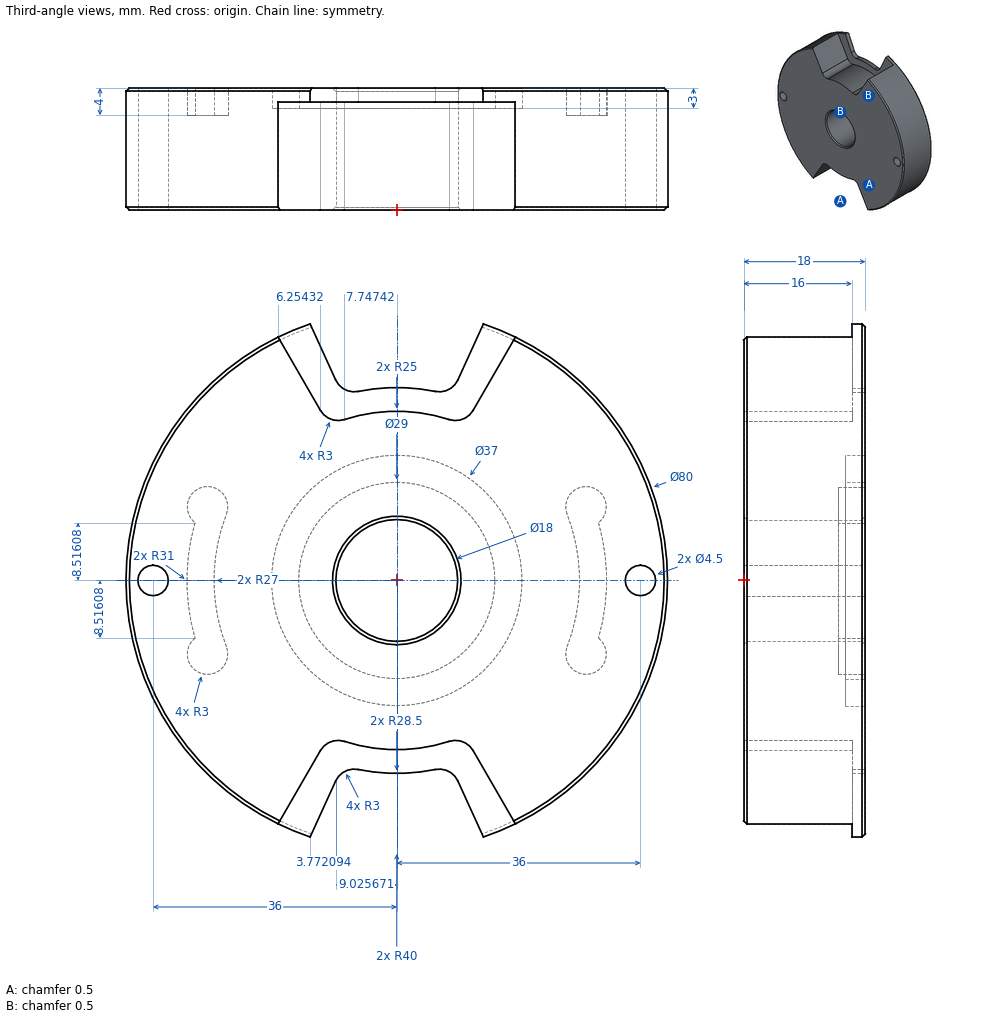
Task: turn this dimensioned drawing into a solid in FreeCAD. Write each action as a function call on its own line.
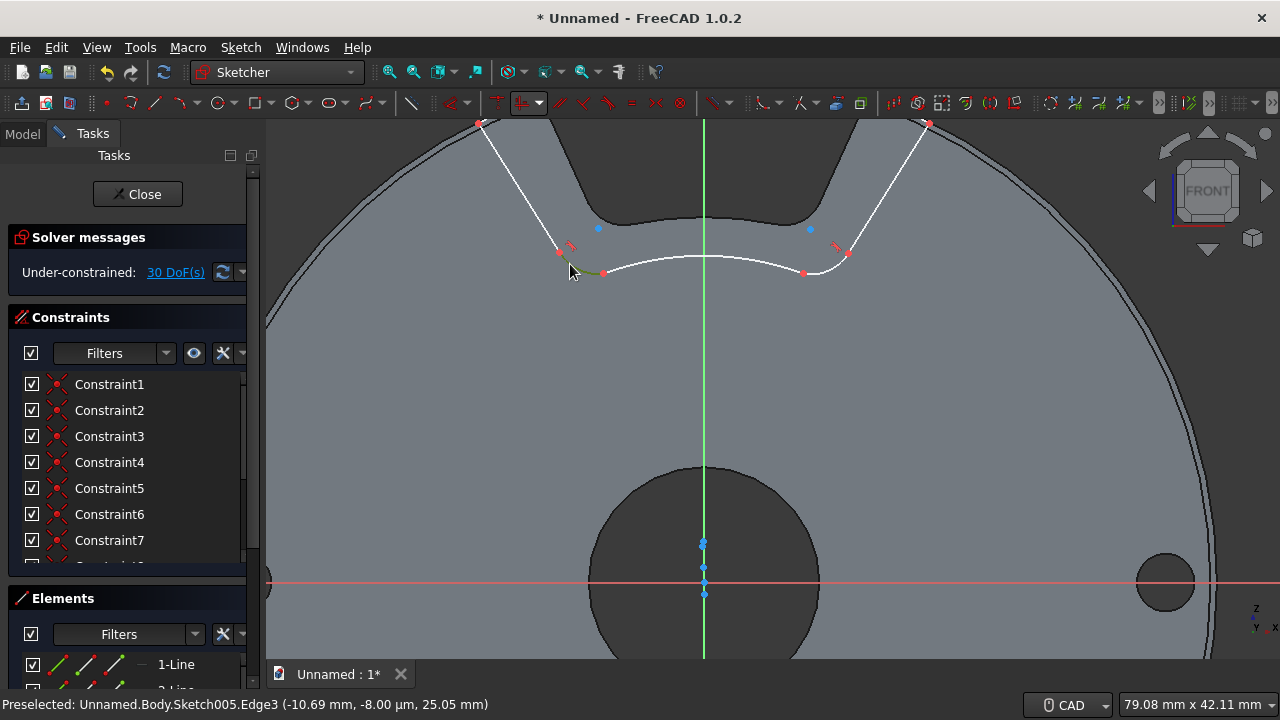
click(744, 259)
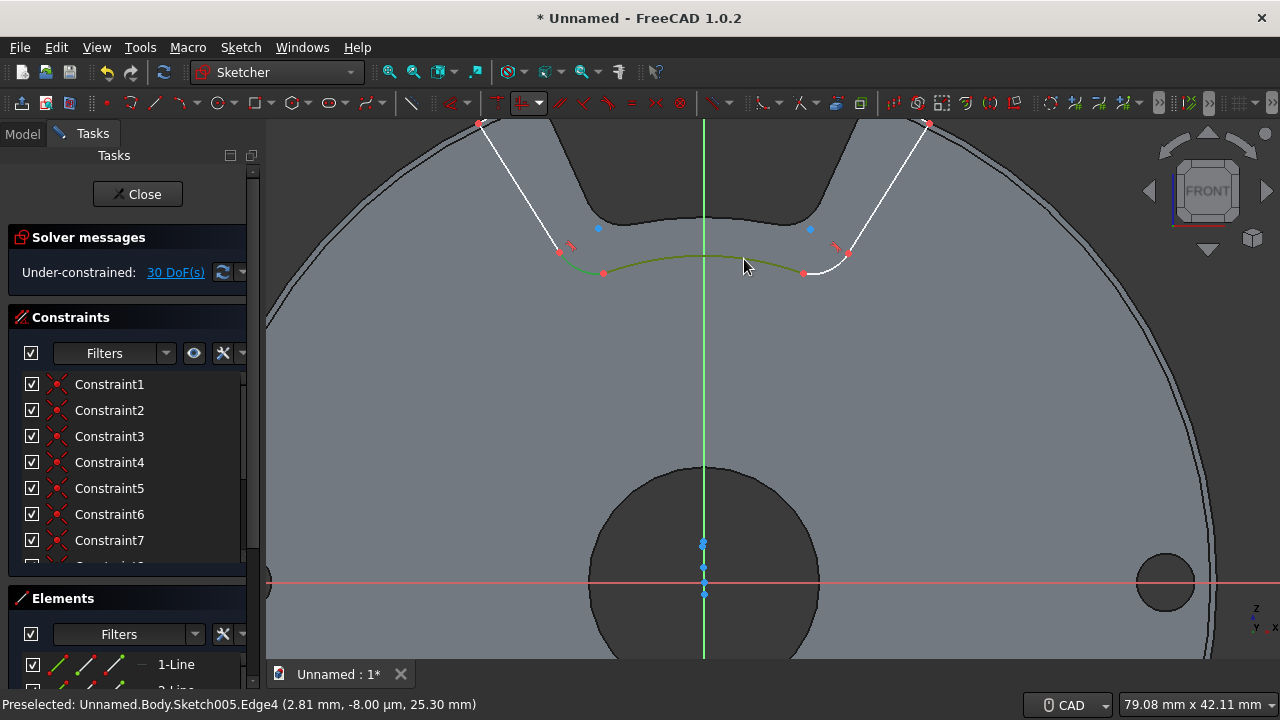
click(608, 104)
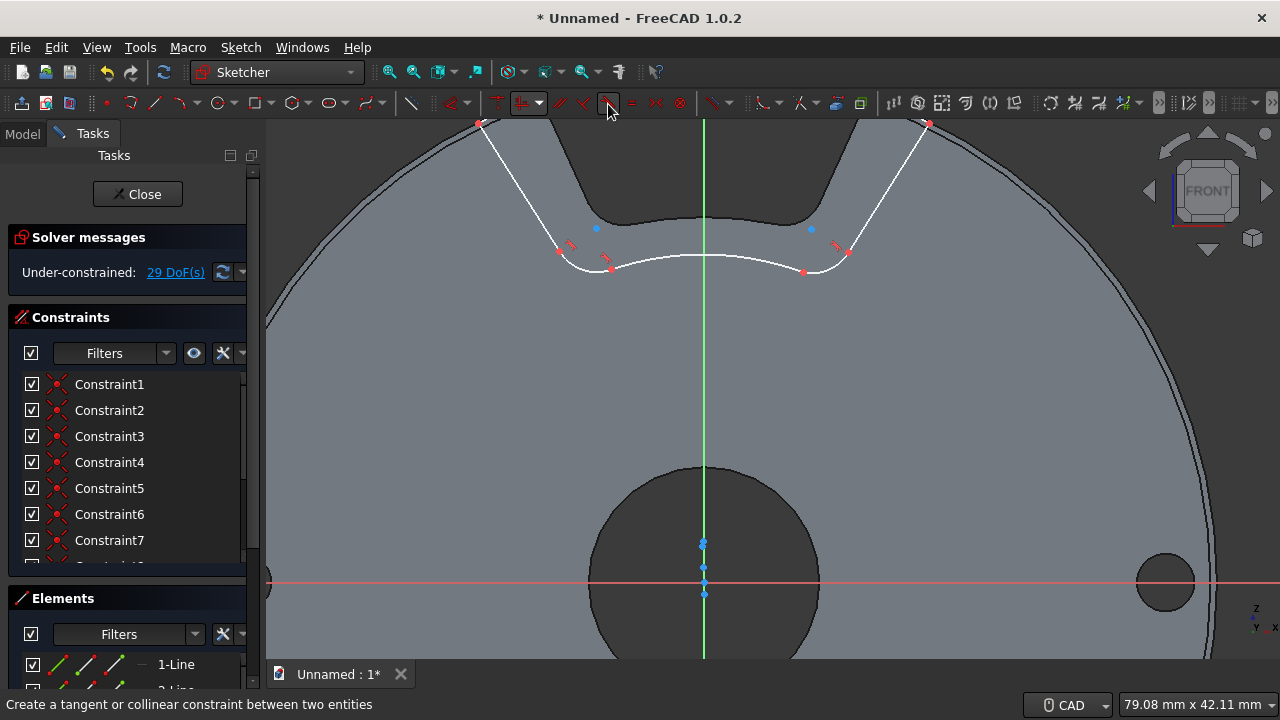
click(746, 258)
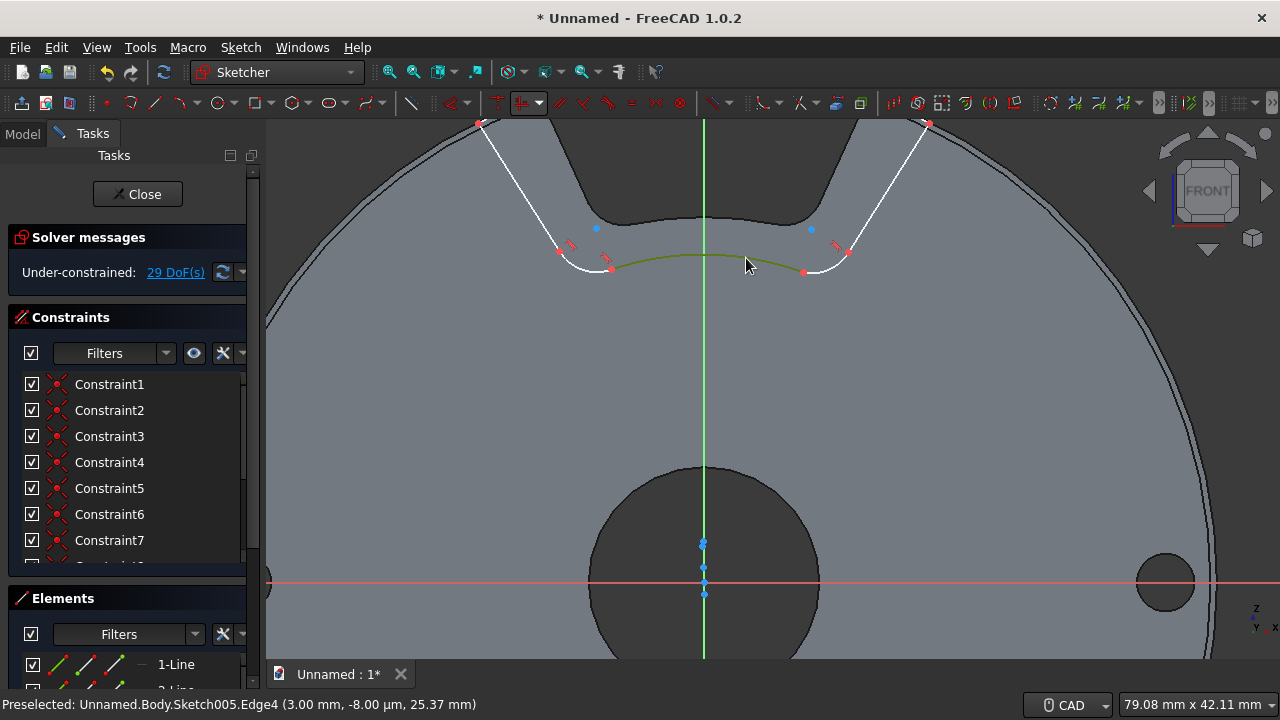
click(819, 273)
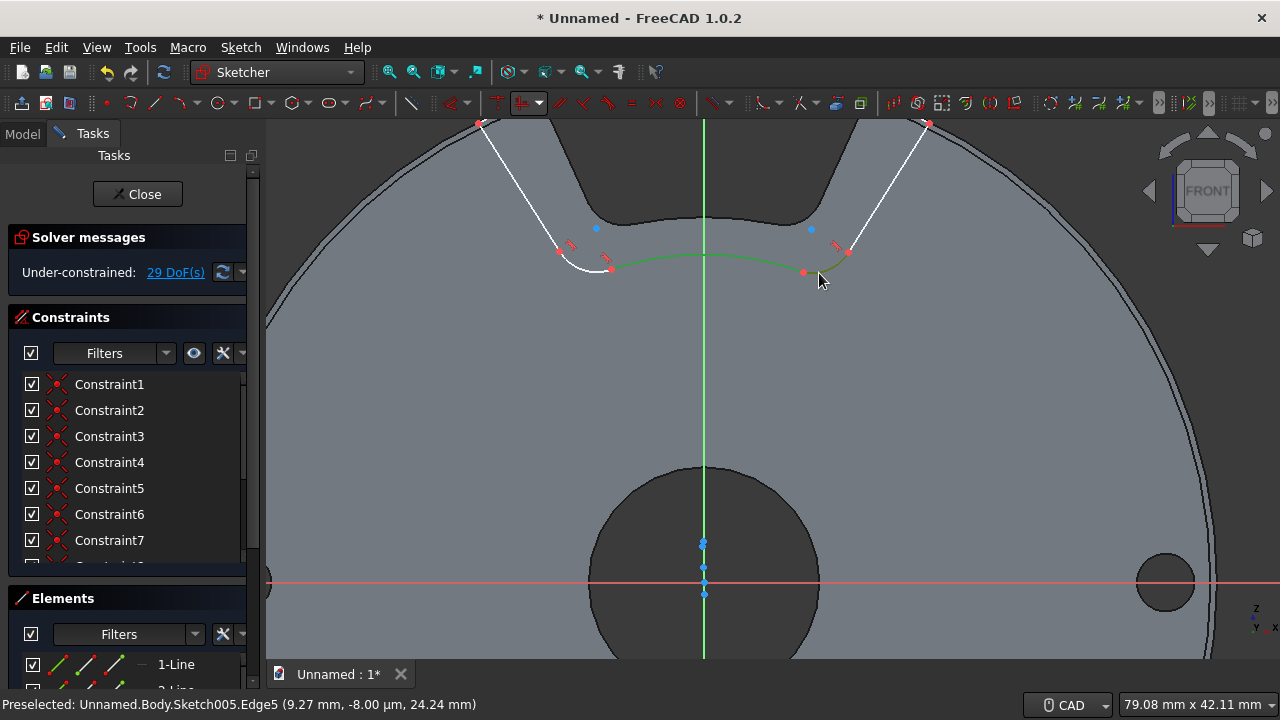
click(608, 104)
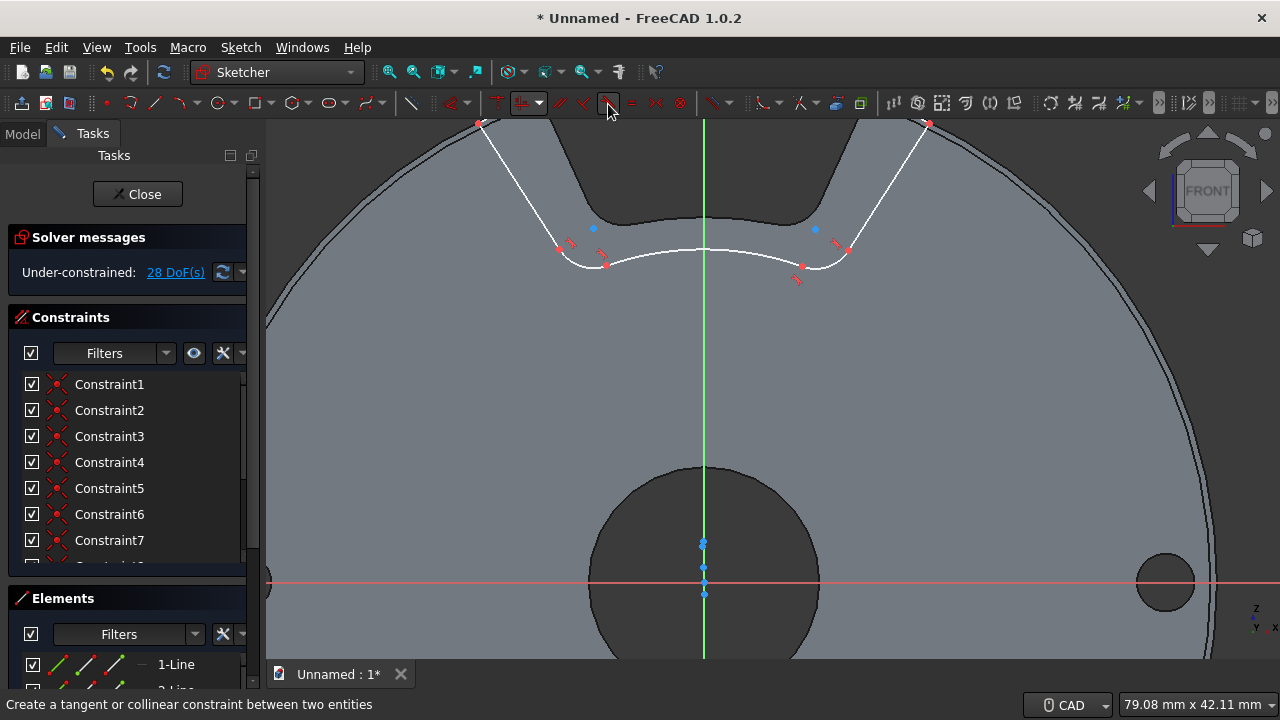
scroll(705, 276, down, 5)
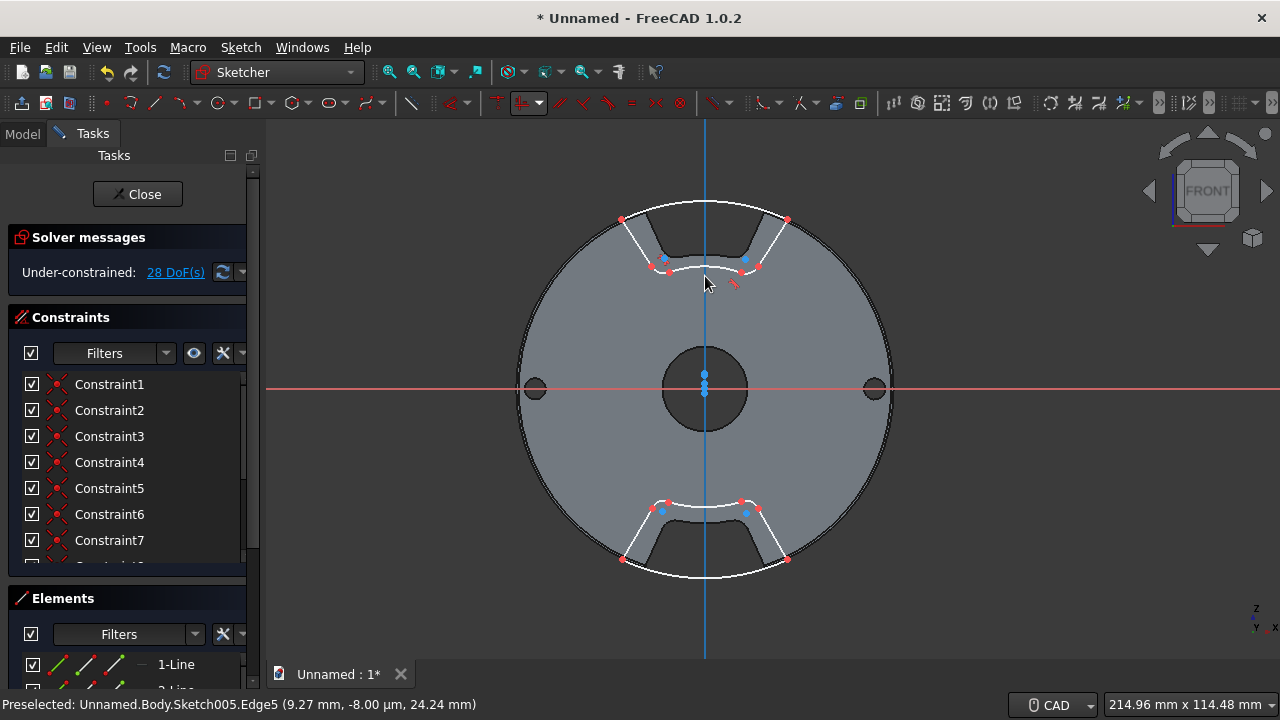
click(778, 545)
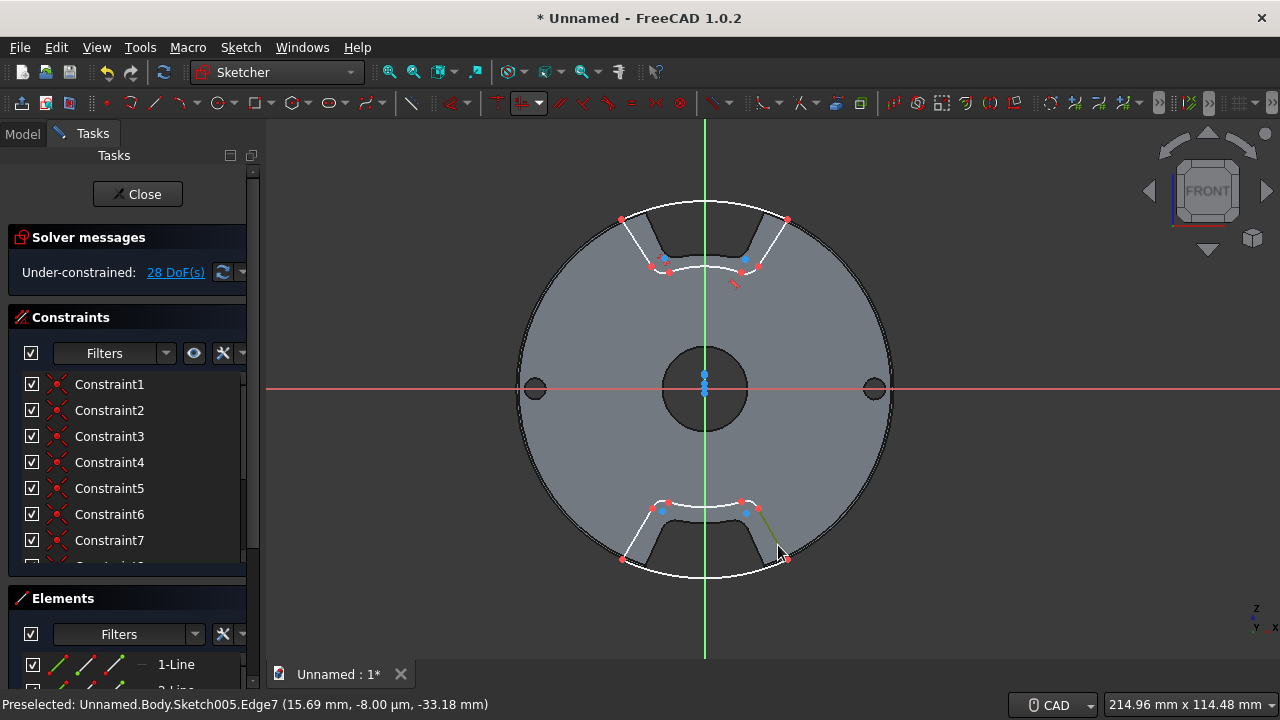
scroll(751, 502, up, 2)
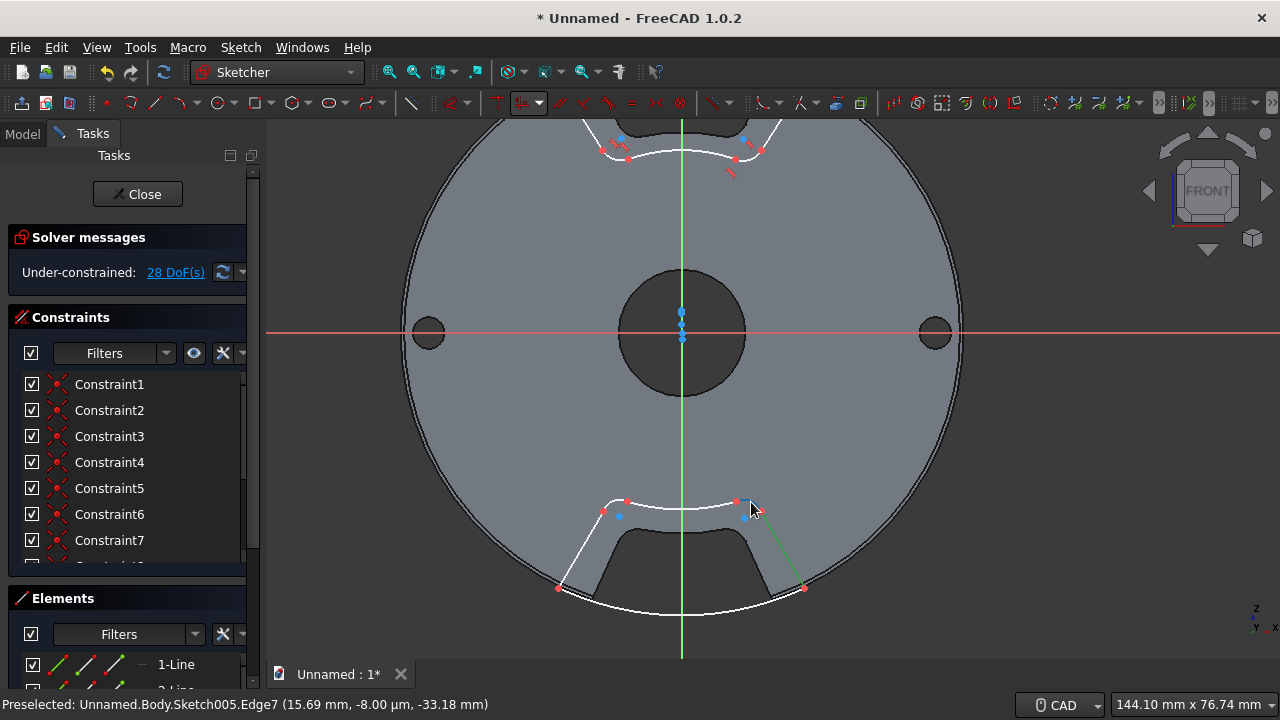
click(751, 501)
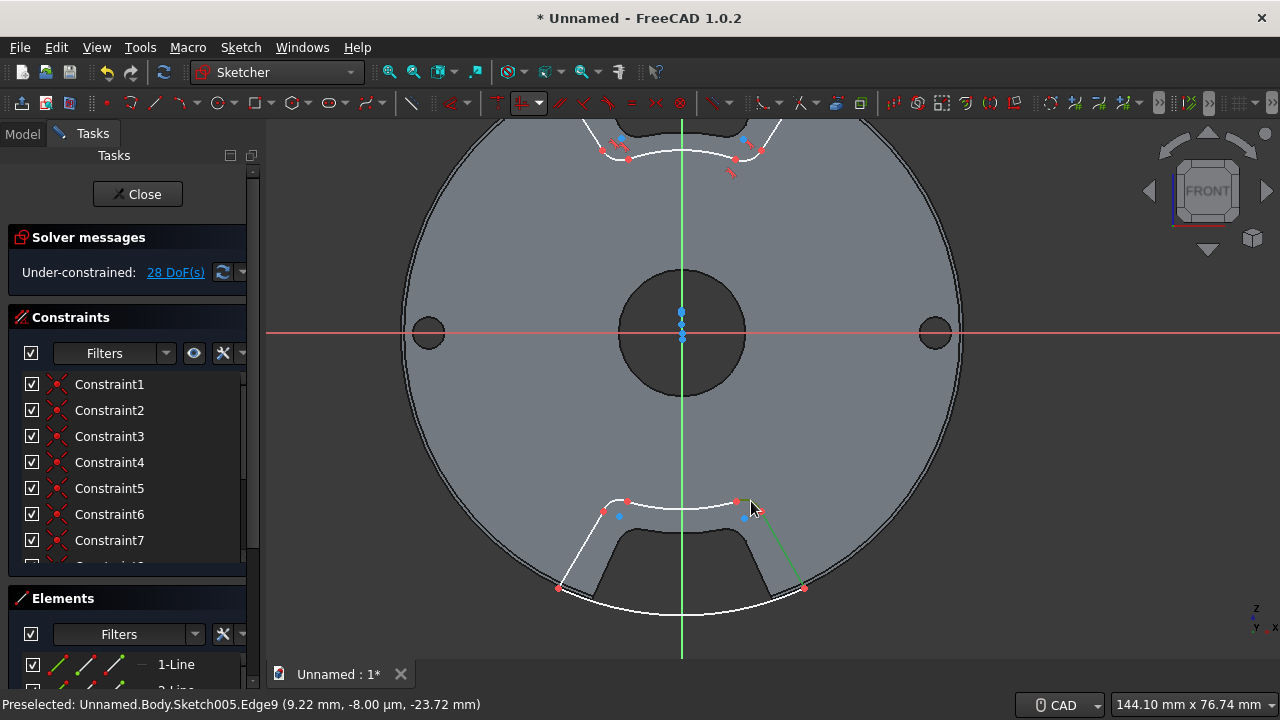
click(608, 104)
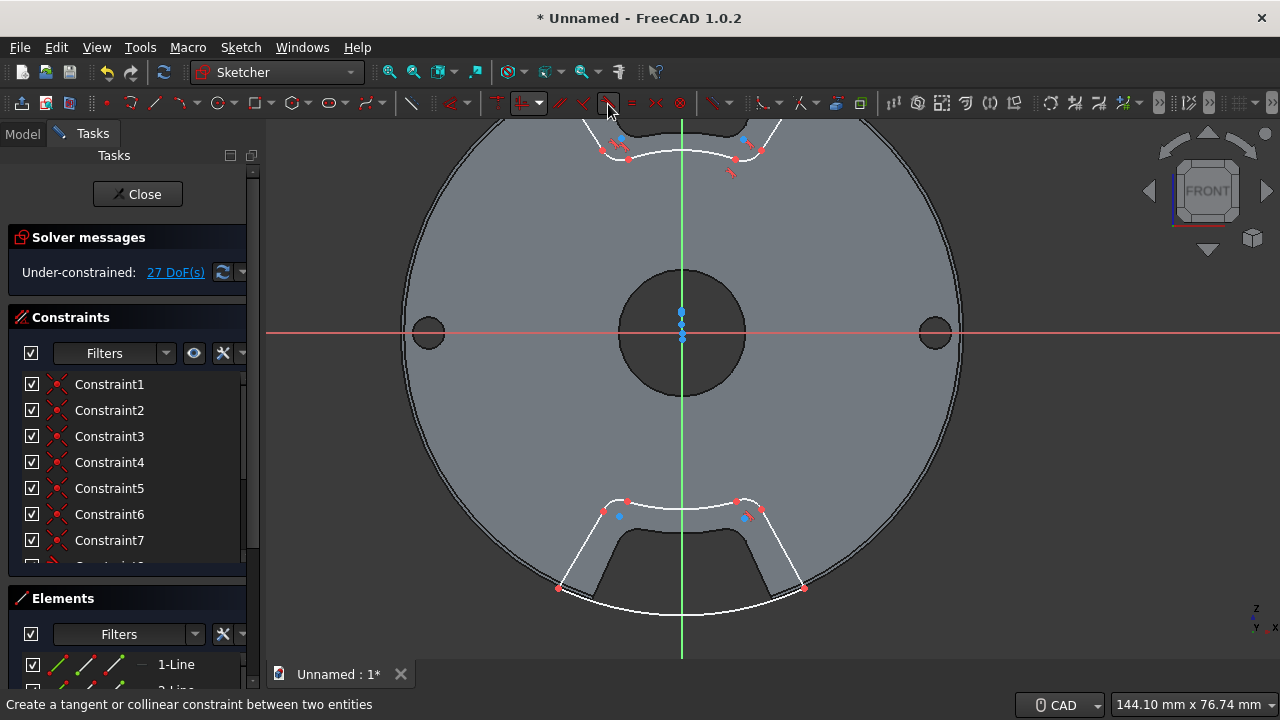
click(590, 535)